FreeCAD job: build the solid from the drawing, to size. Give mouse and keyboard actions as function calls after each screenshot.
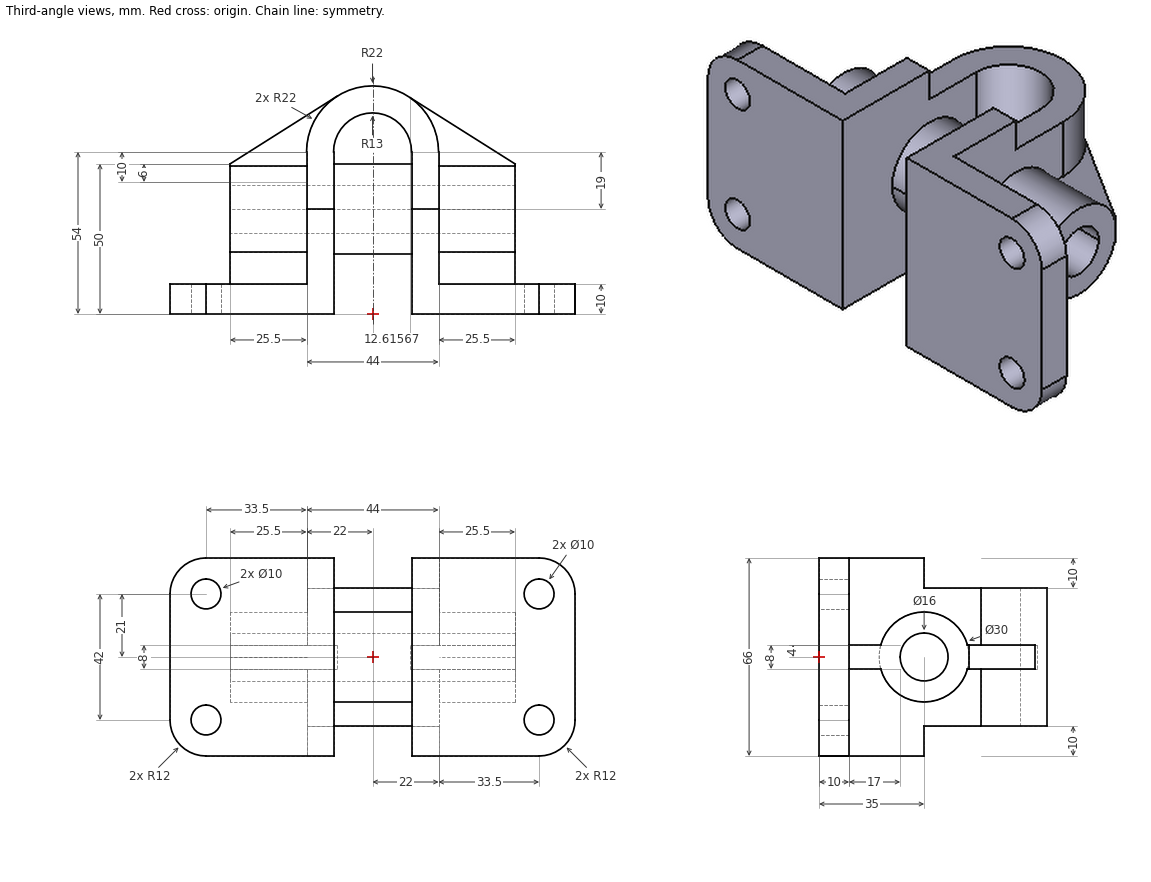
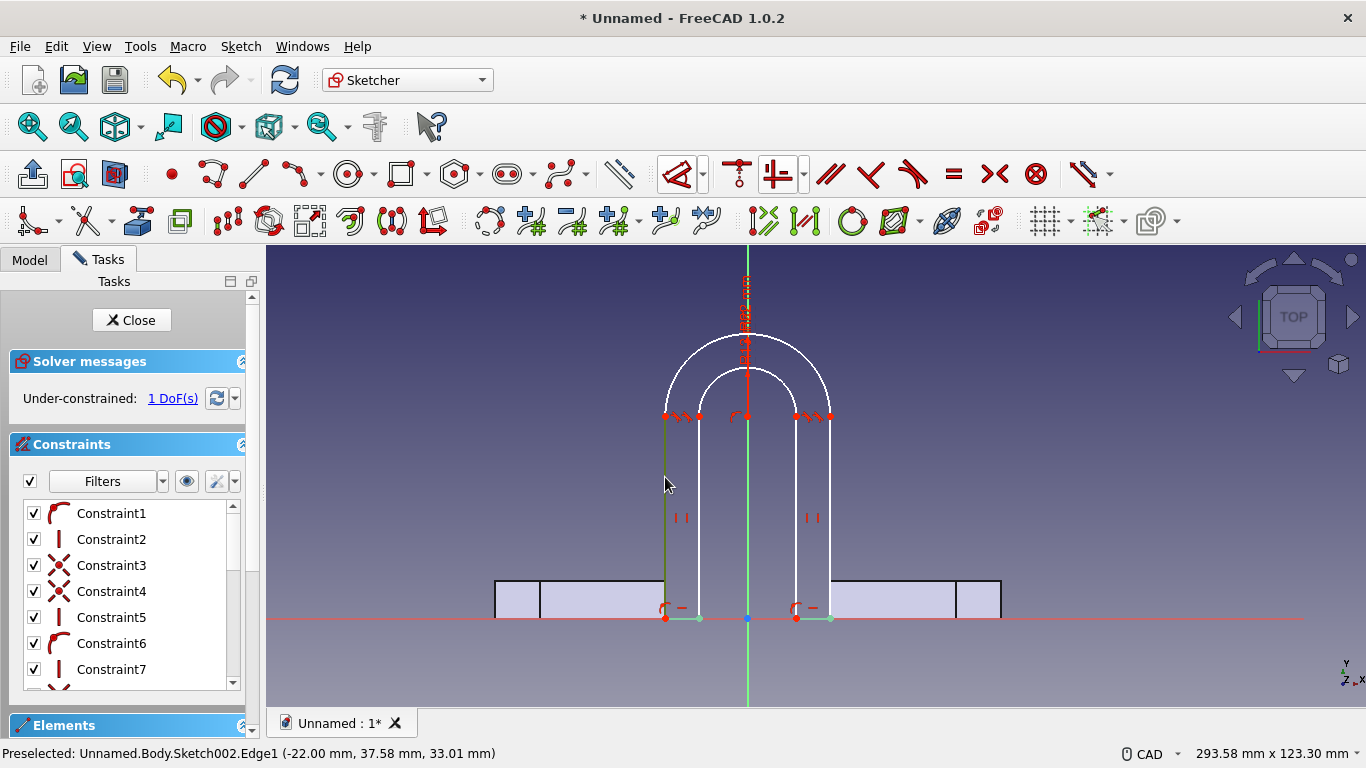
key(i)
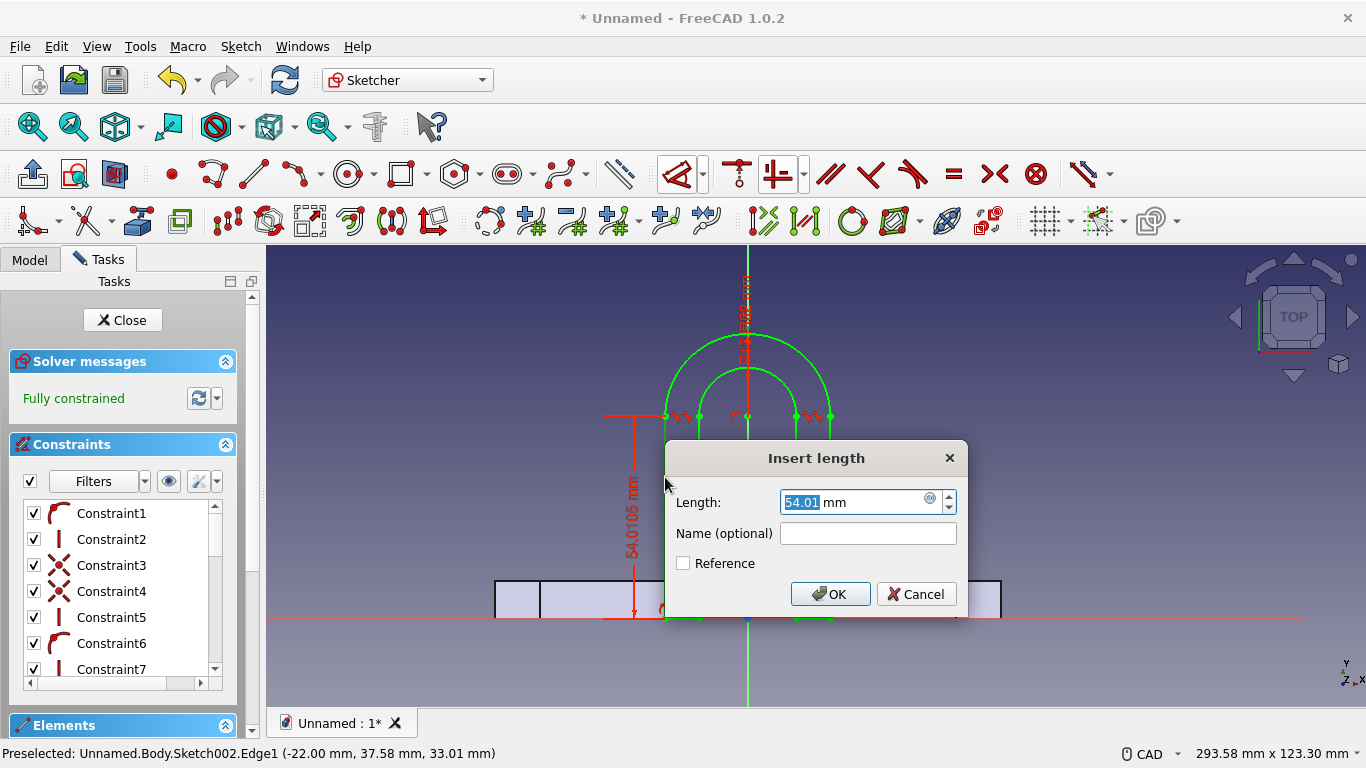
text(54)
key(Return)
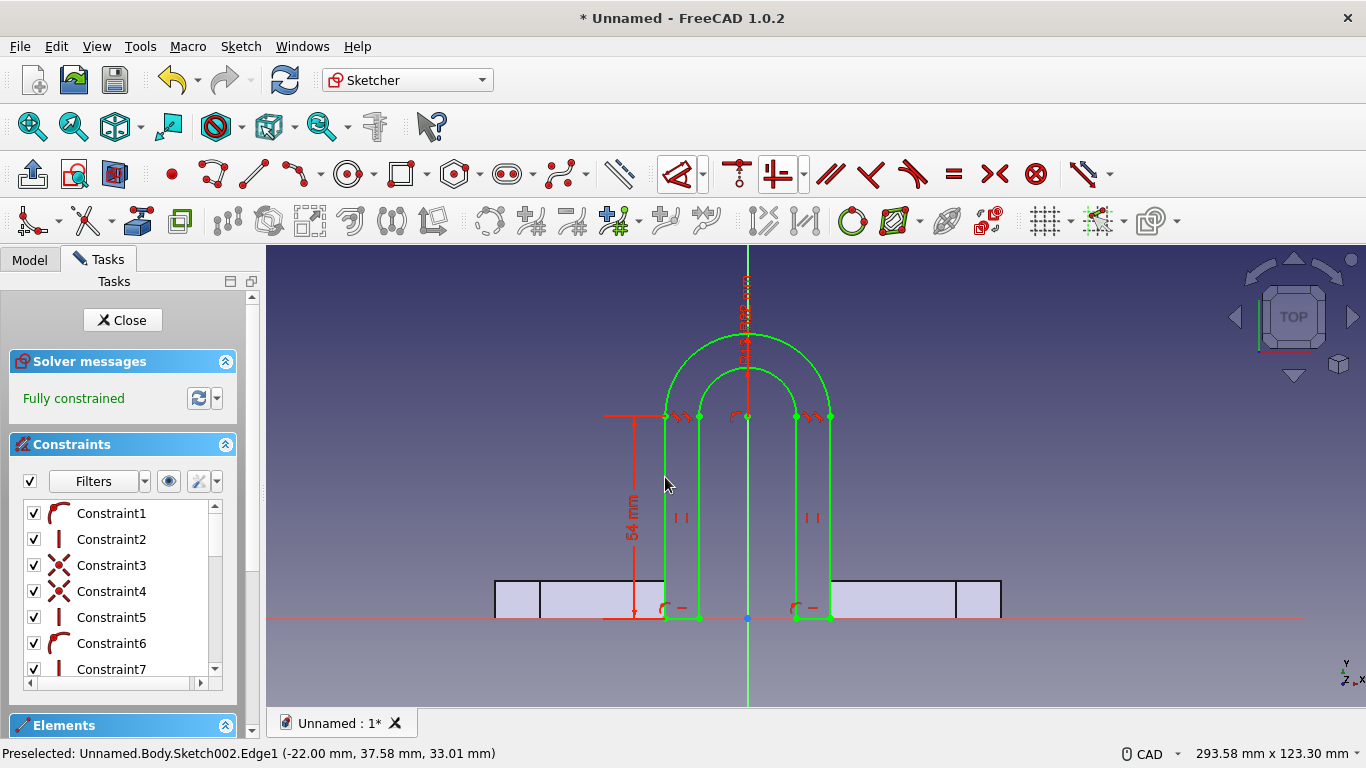
click(123, 320)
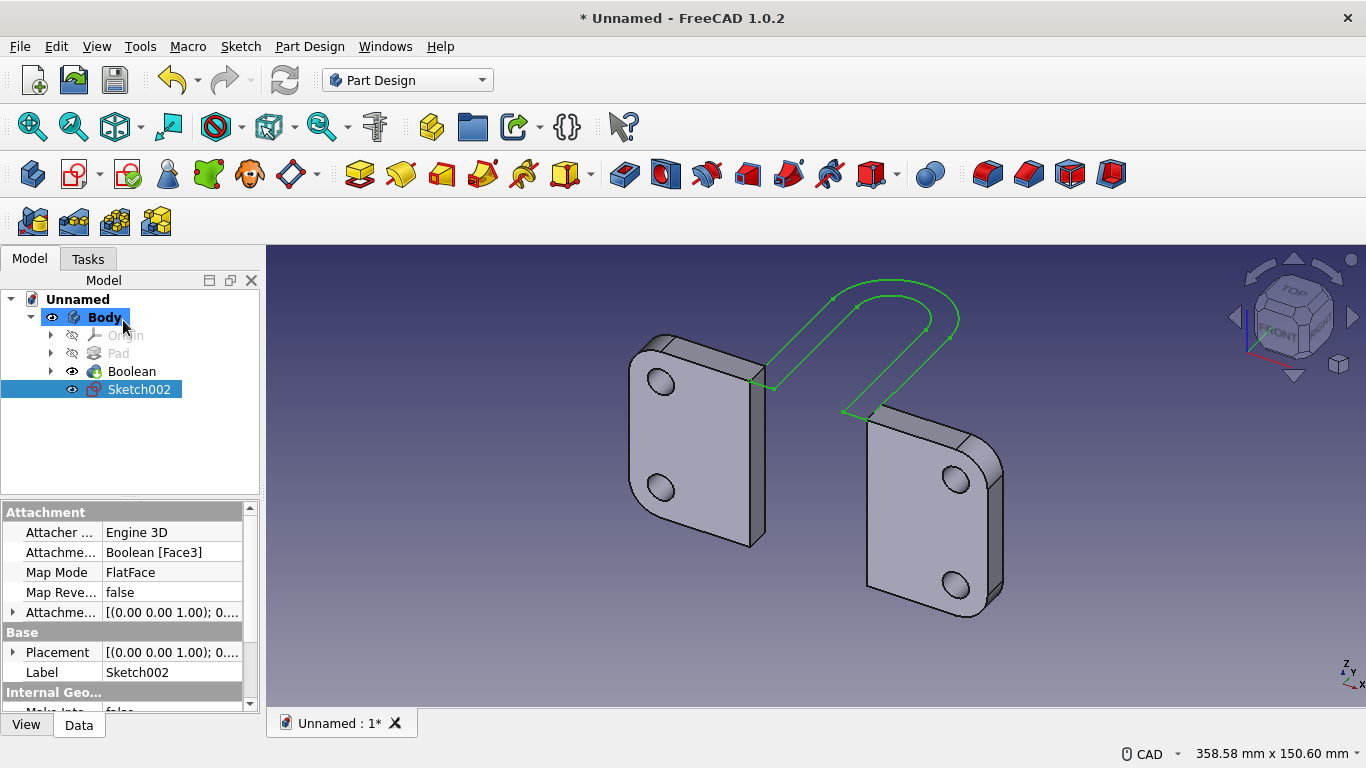
click(360, 174)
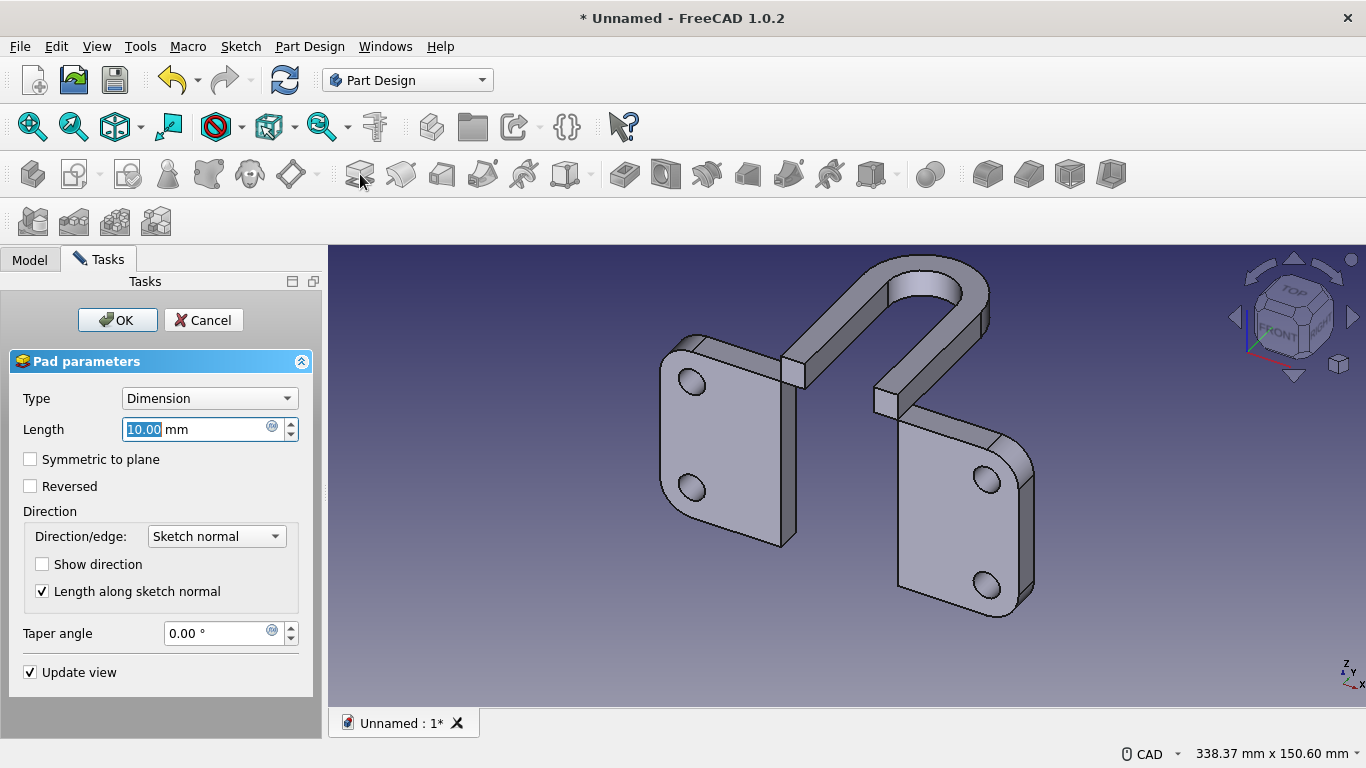
text(66)
key(Tab)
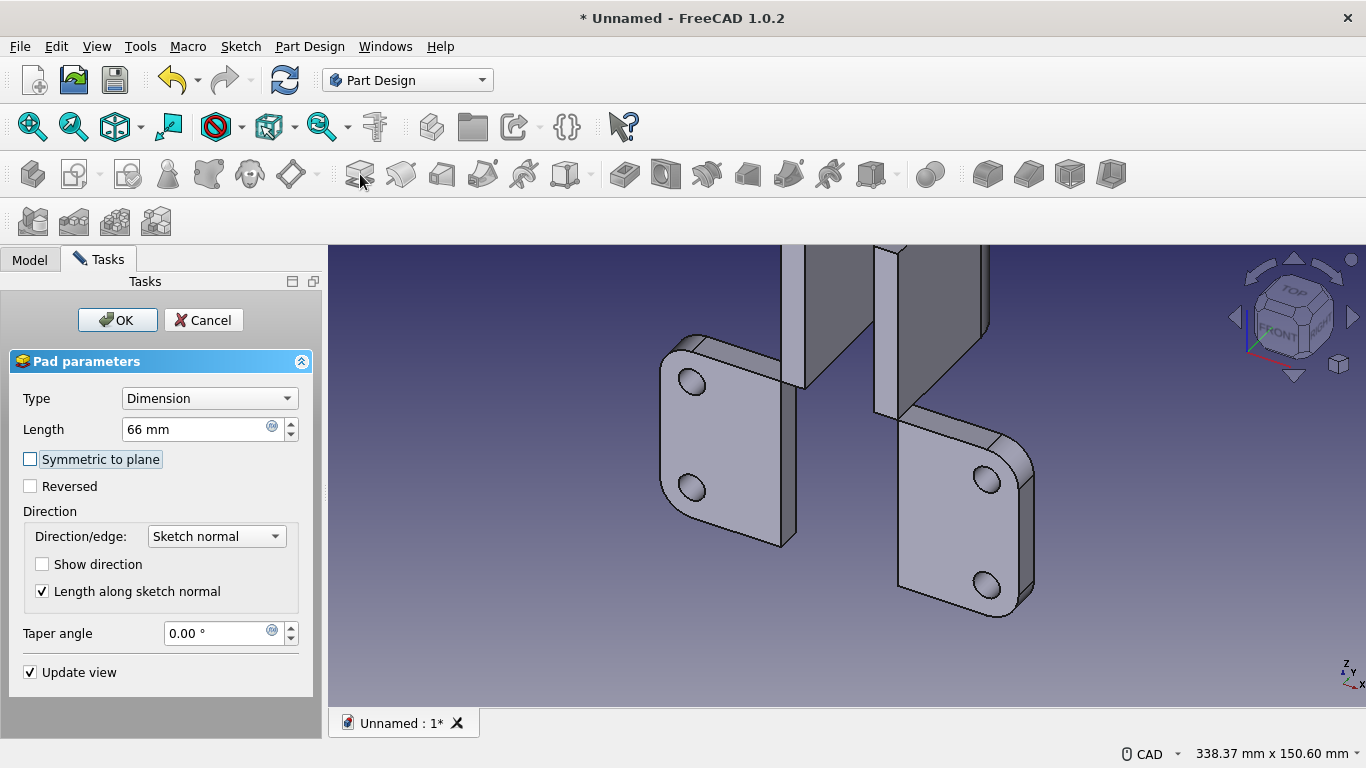
click(31, 486)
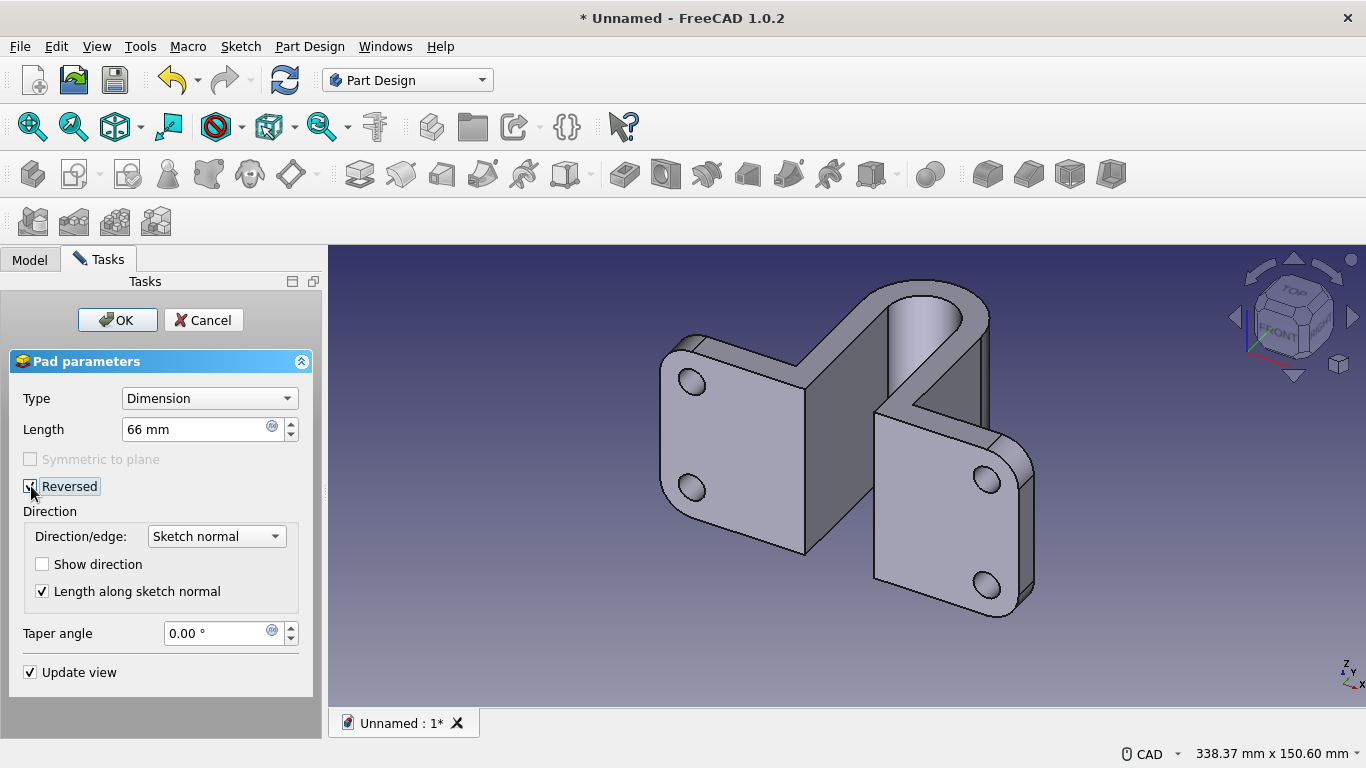
click(118, 320)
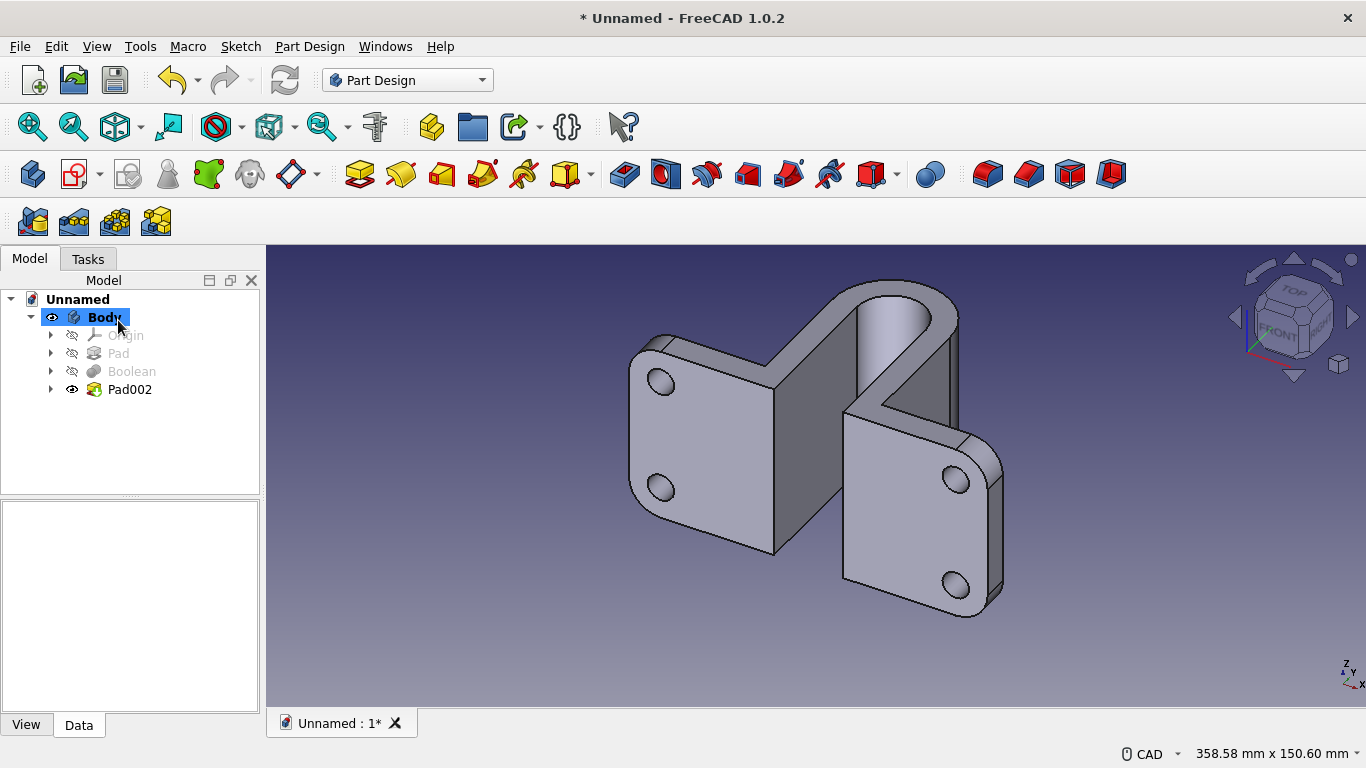
click(33, 128)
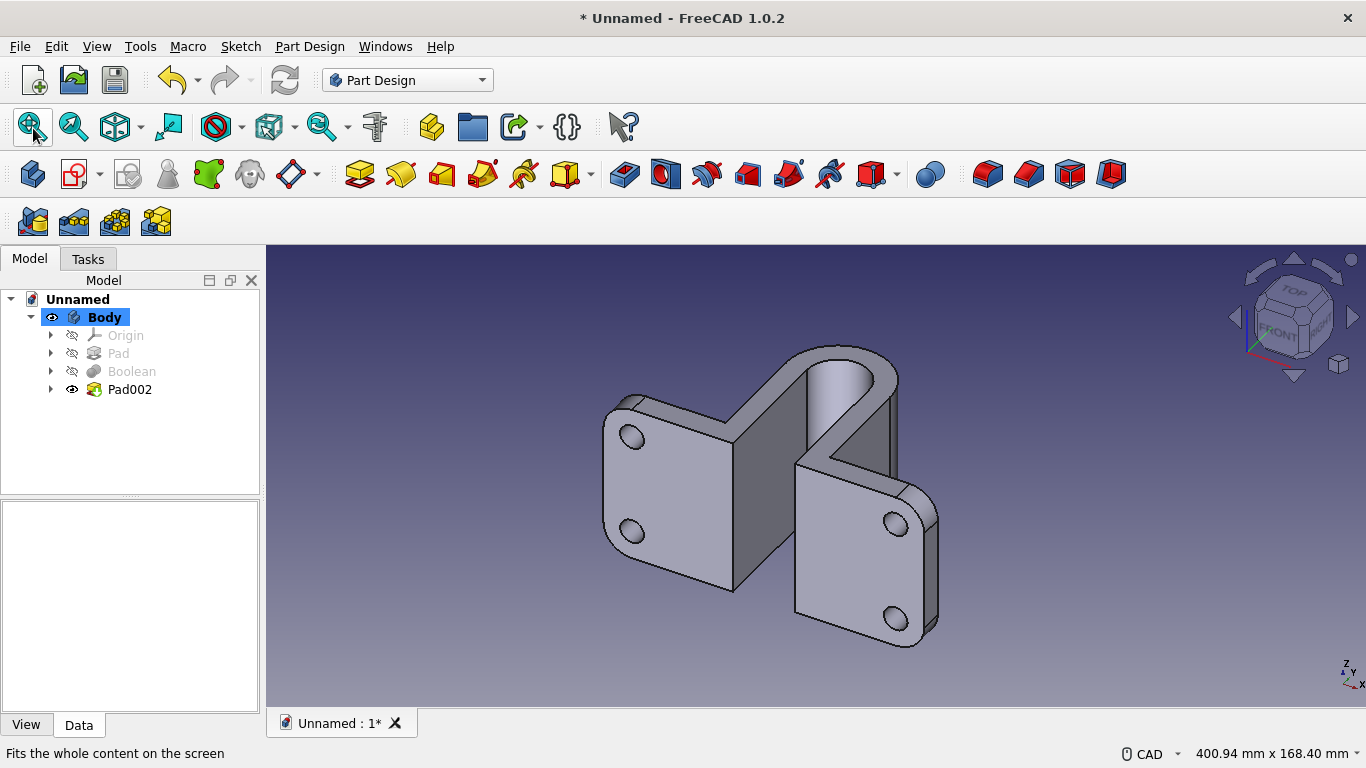
click(696, 420)